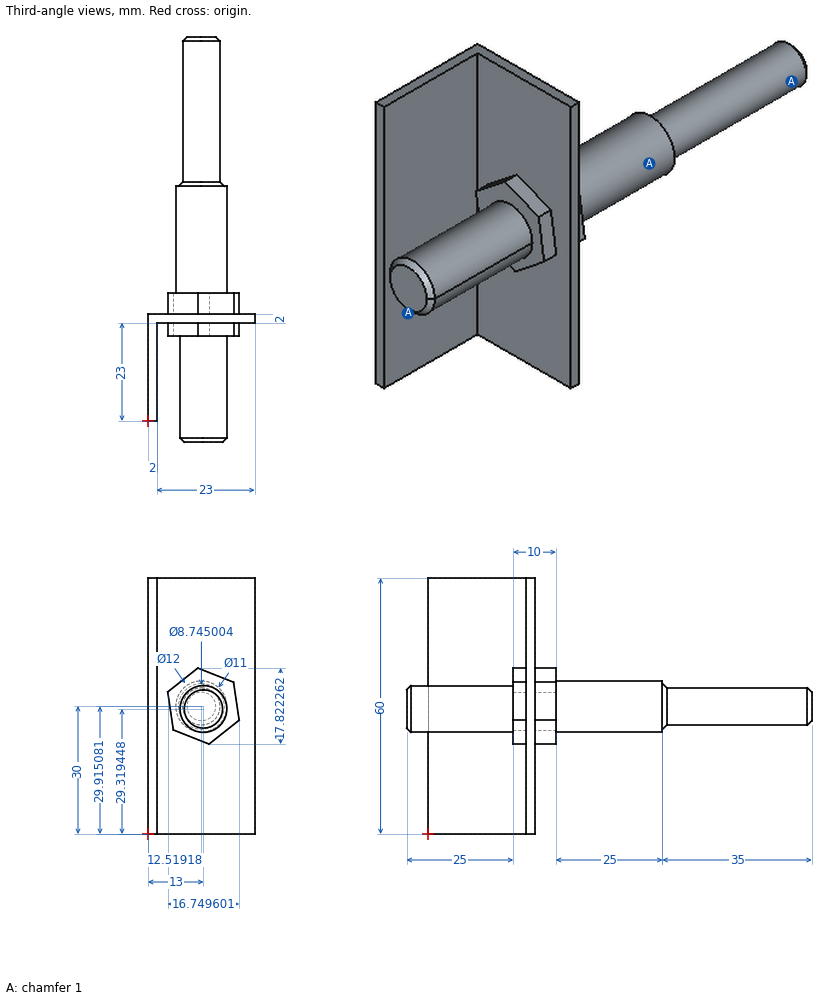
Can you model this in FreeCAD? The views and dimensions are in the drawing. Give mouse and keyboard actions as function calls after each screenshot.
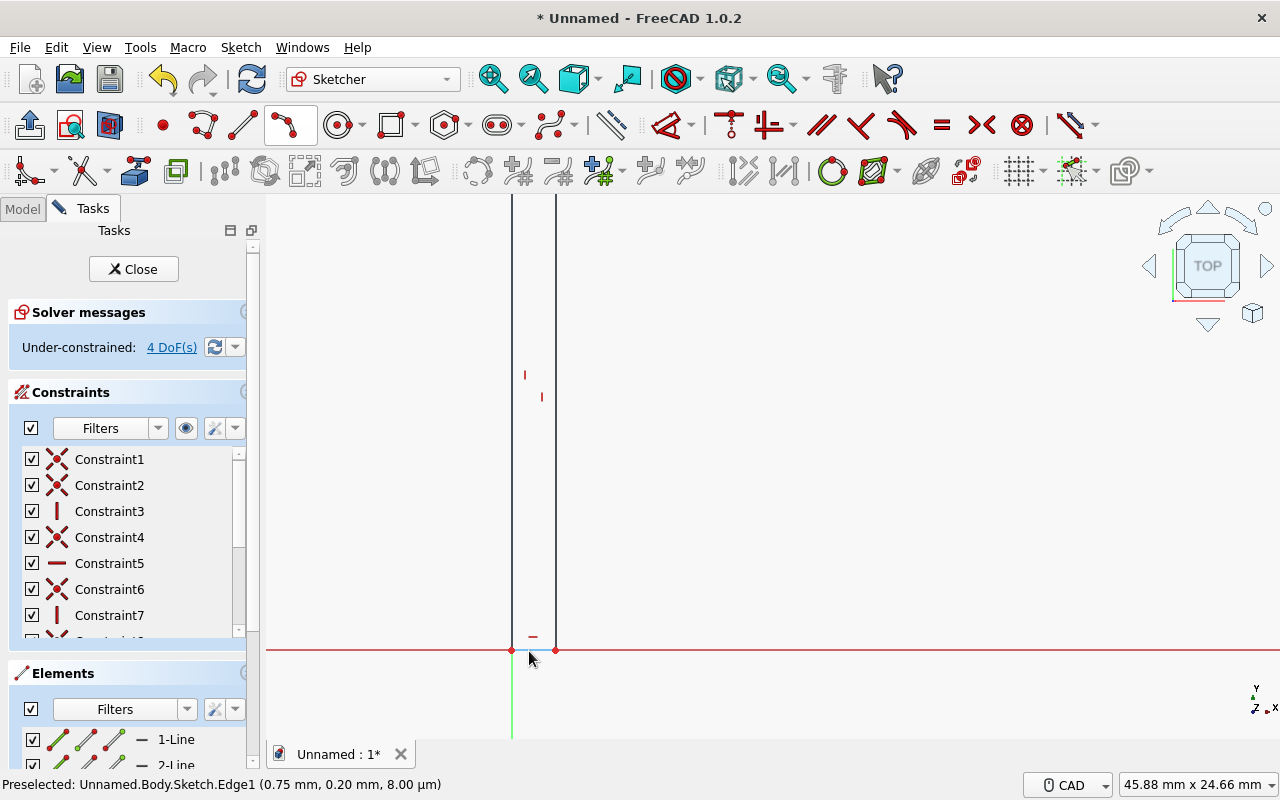
click(529, 650)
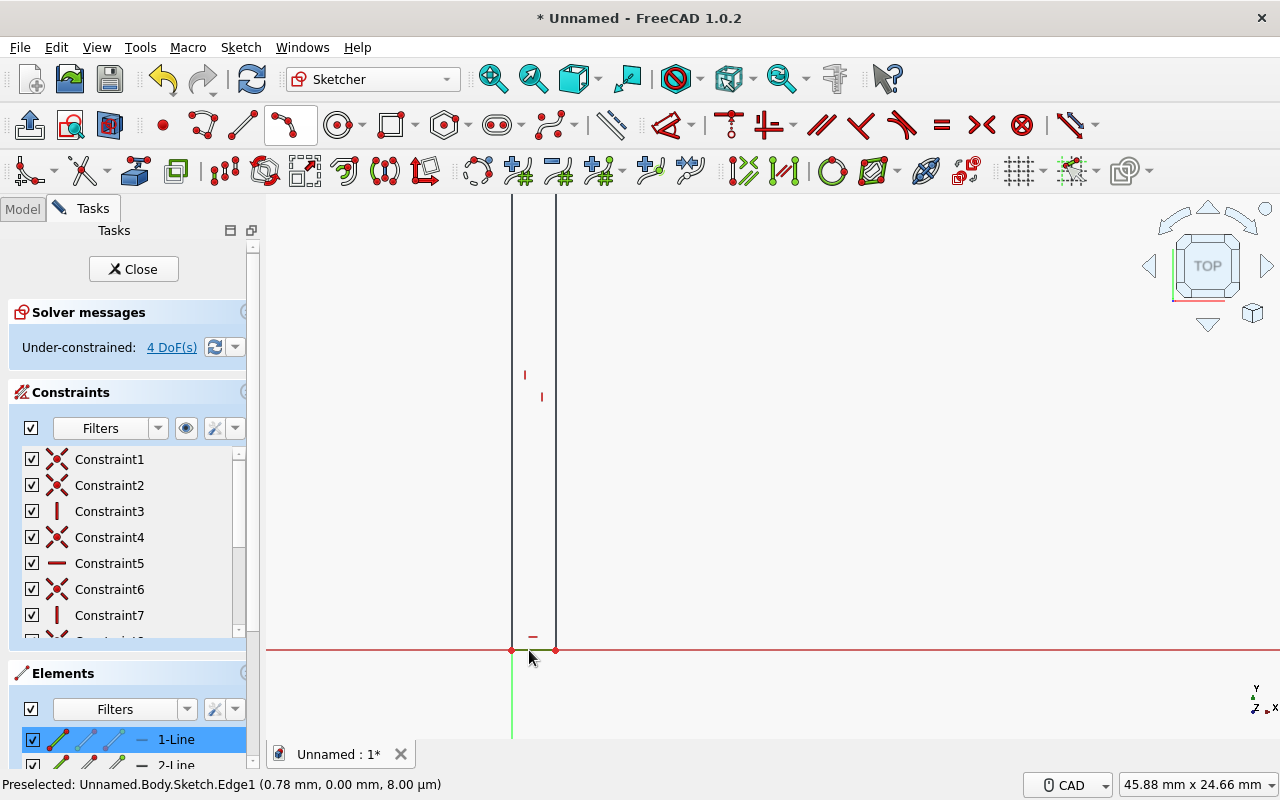
key(l)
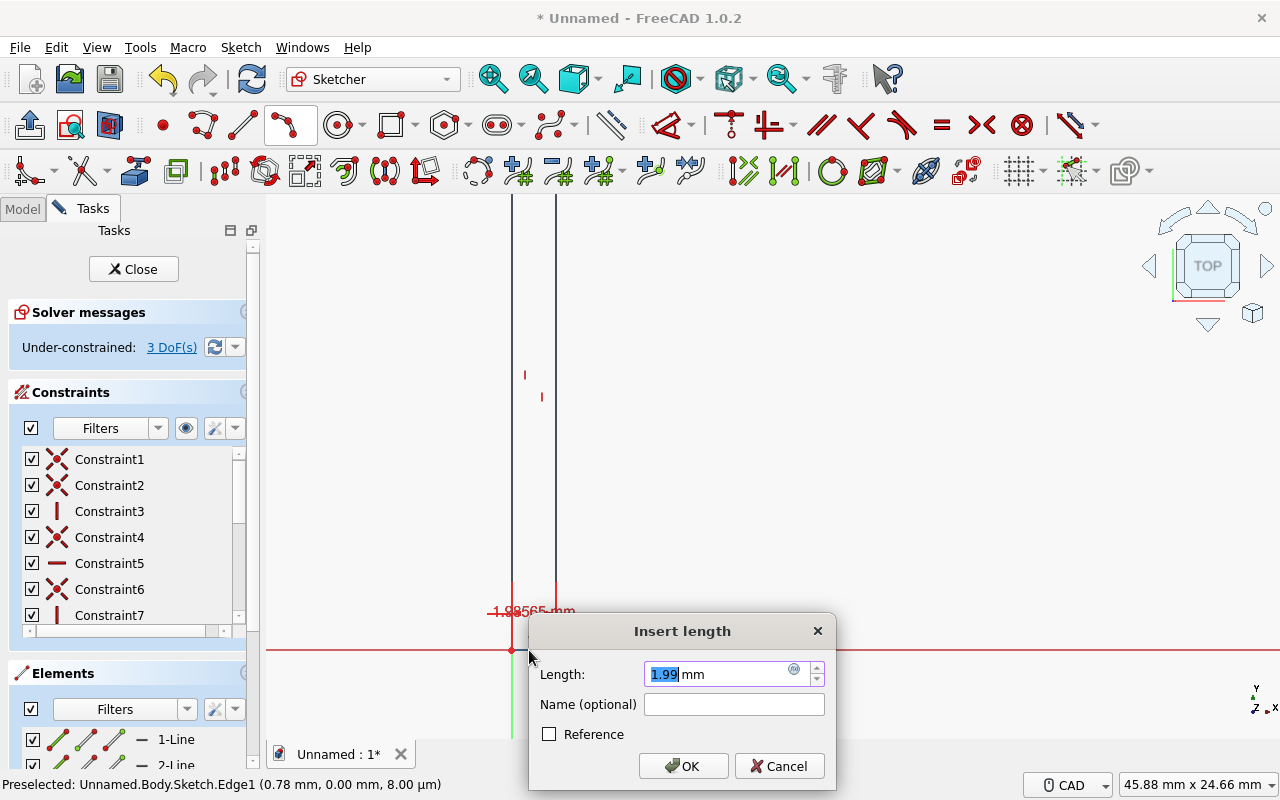
text(2)
key(Return)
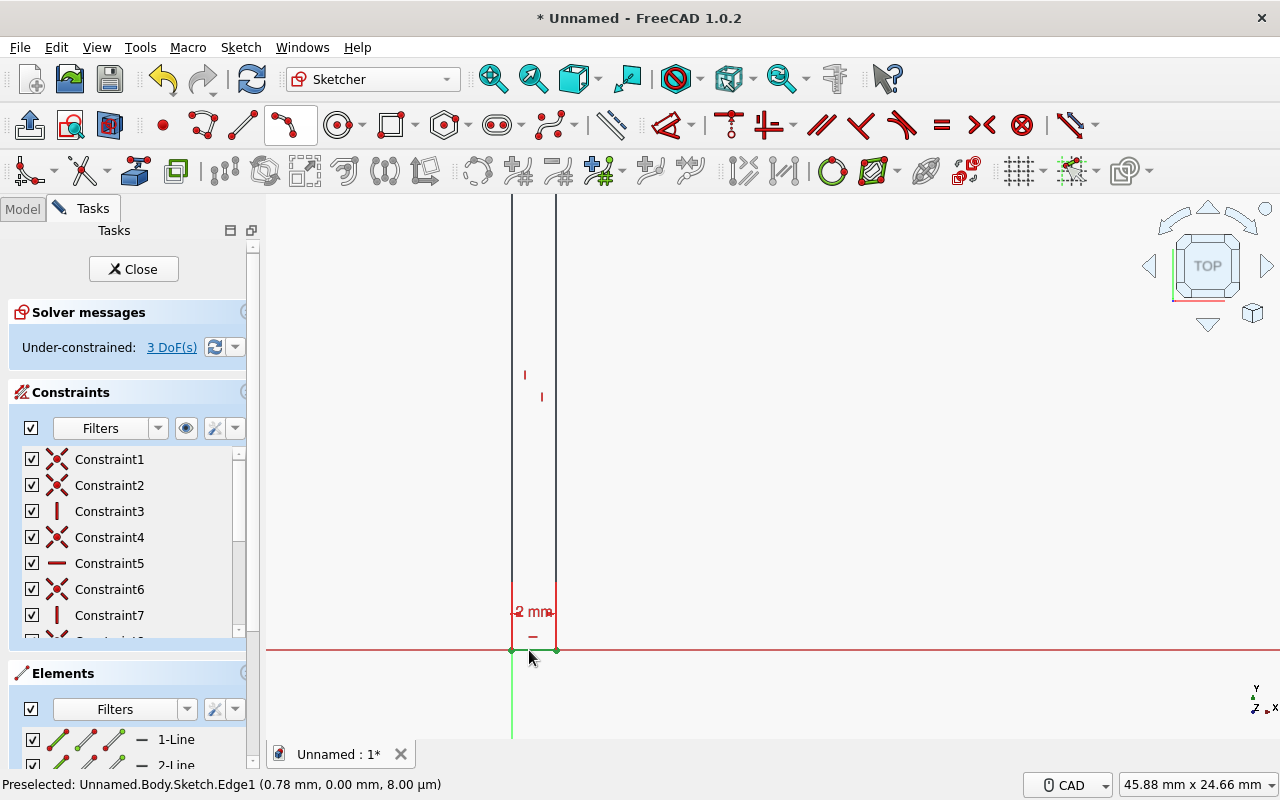
scroll(535, 655, down, 2)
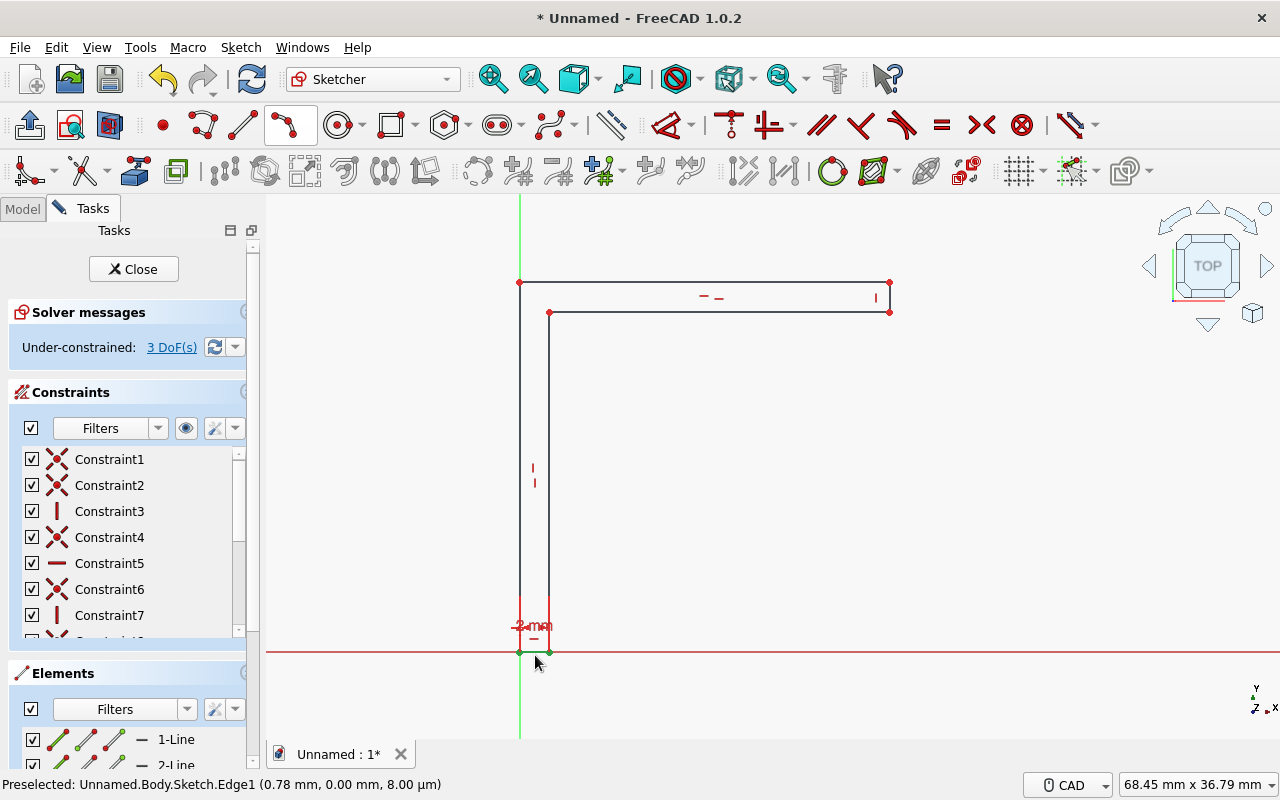
scroll(890, 303, up, 3)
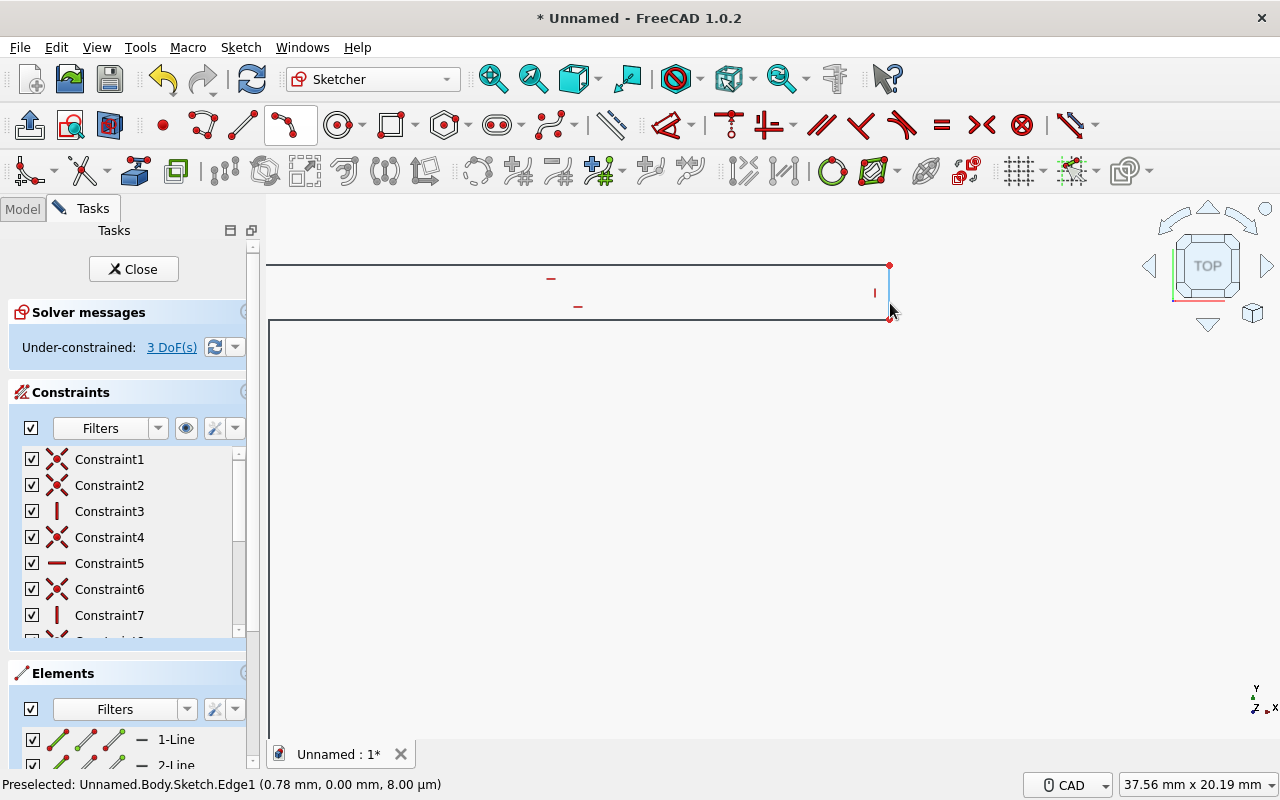
click(889, 303)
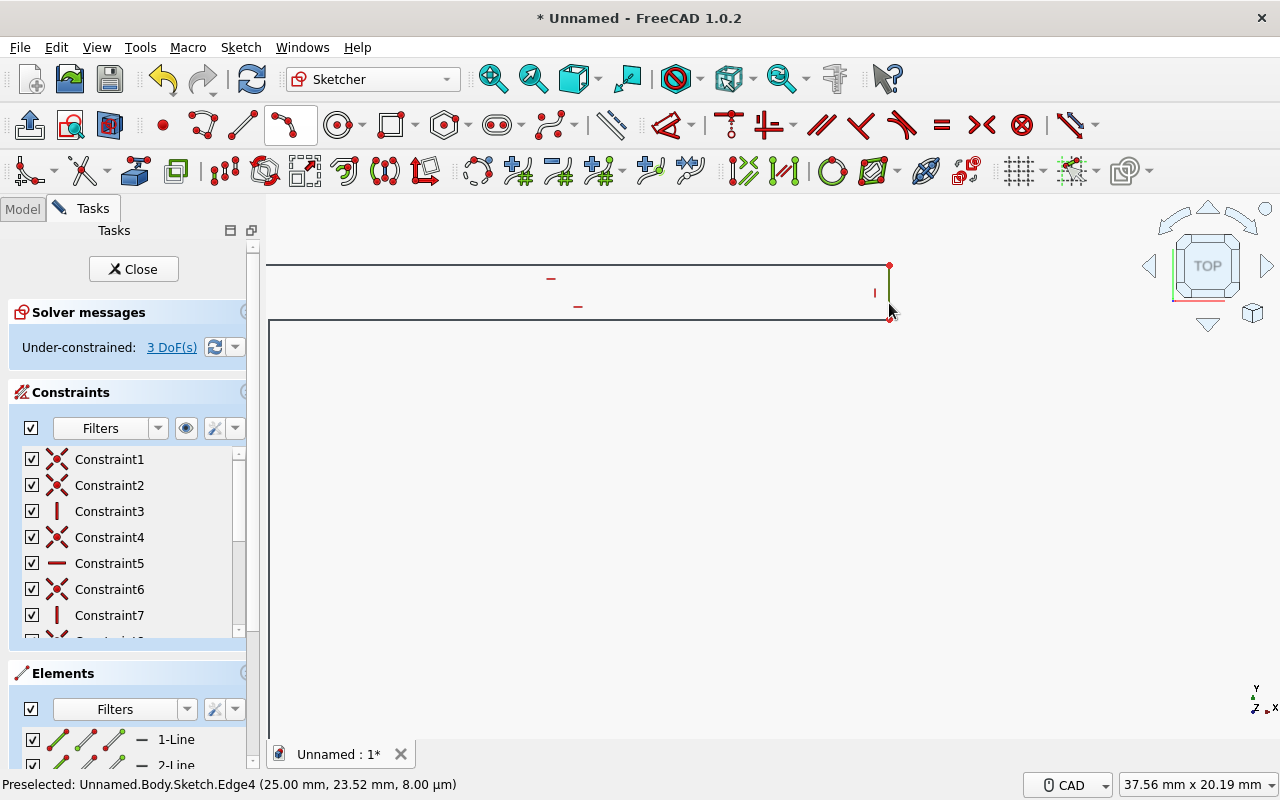
key(i)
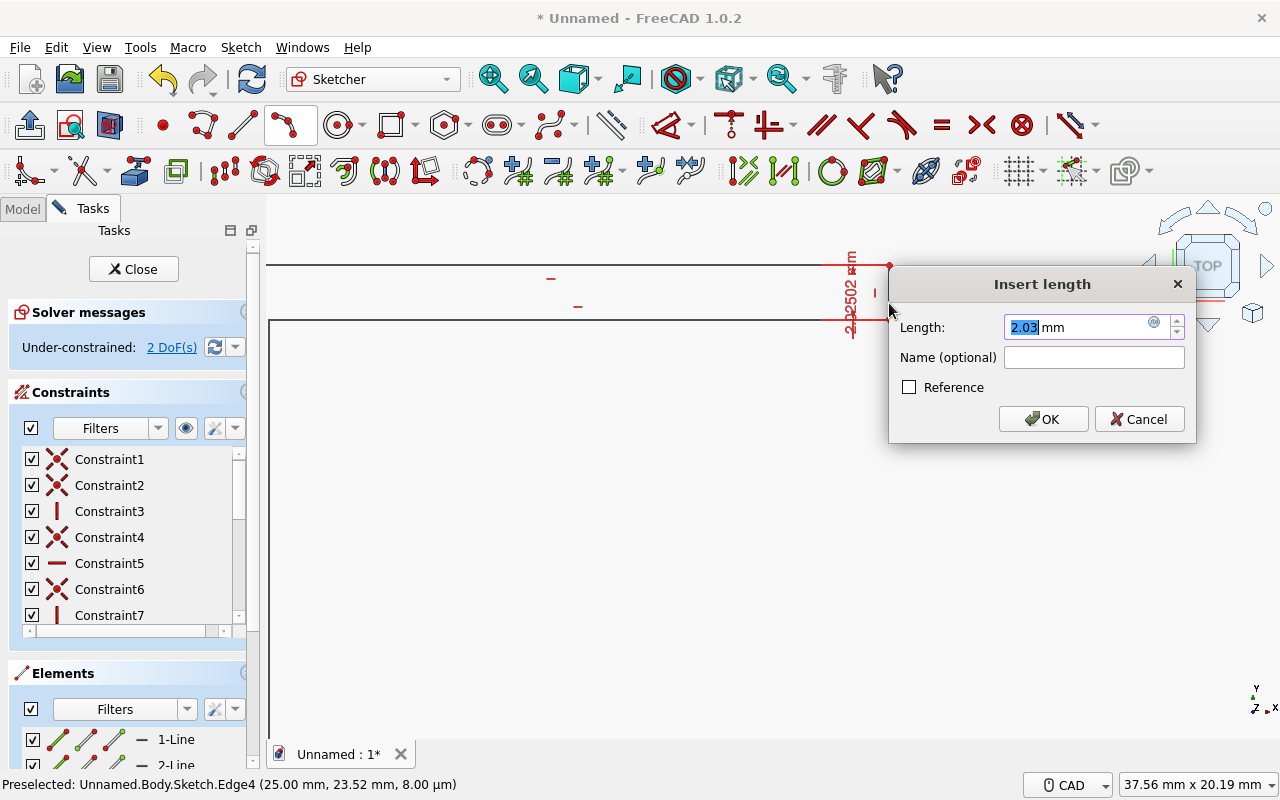
text(2)
key(Return)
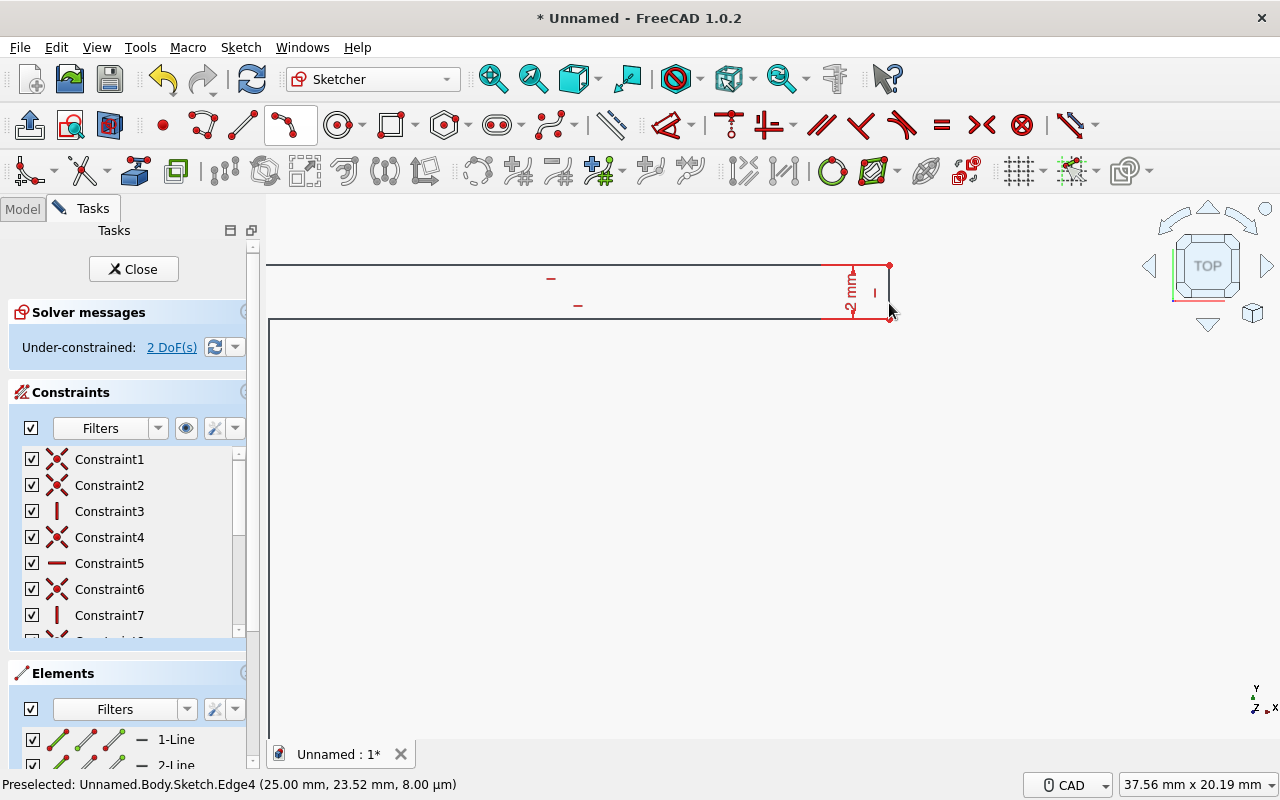
scroll(890, 302, down, 3)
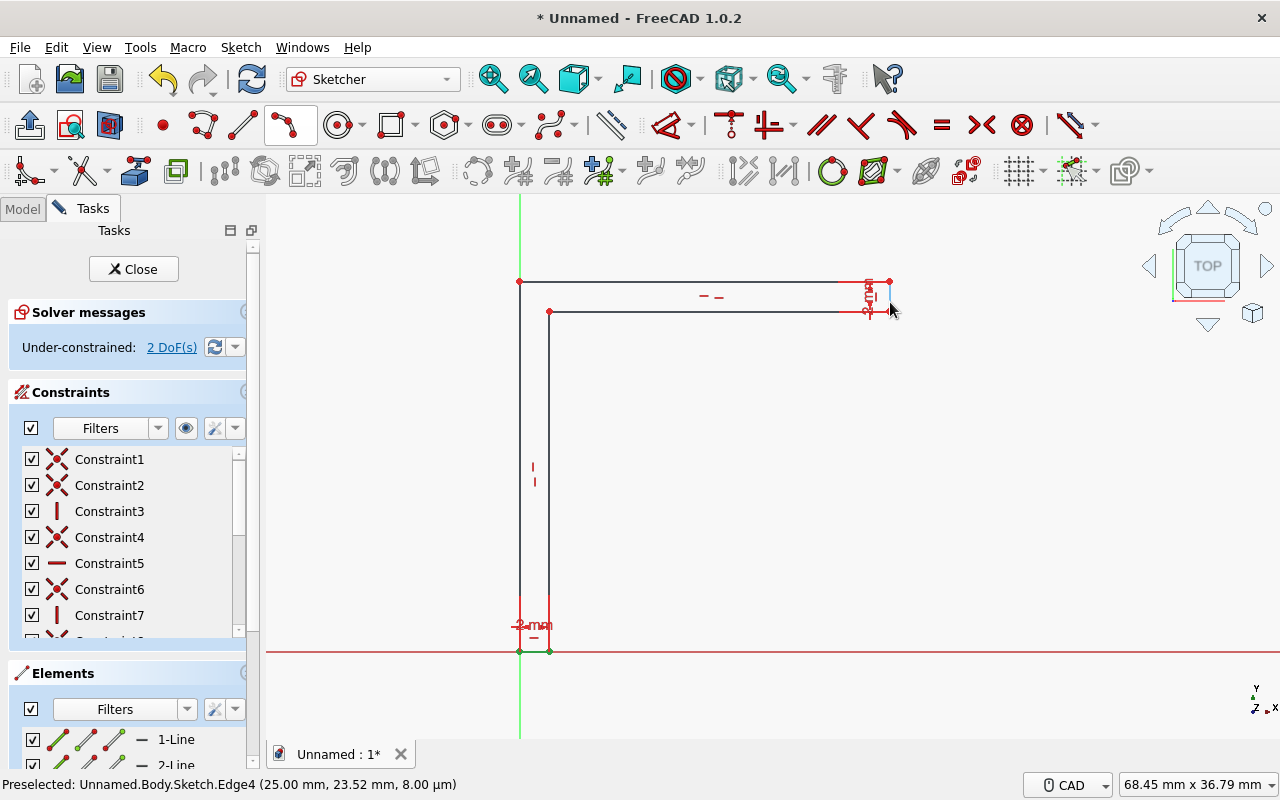
click(549, 550)